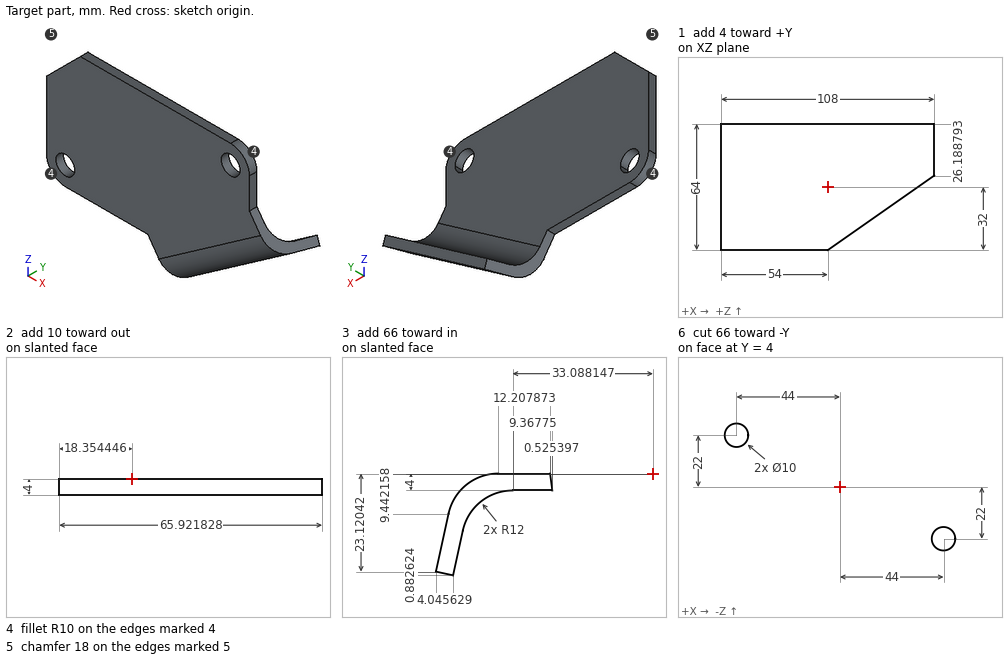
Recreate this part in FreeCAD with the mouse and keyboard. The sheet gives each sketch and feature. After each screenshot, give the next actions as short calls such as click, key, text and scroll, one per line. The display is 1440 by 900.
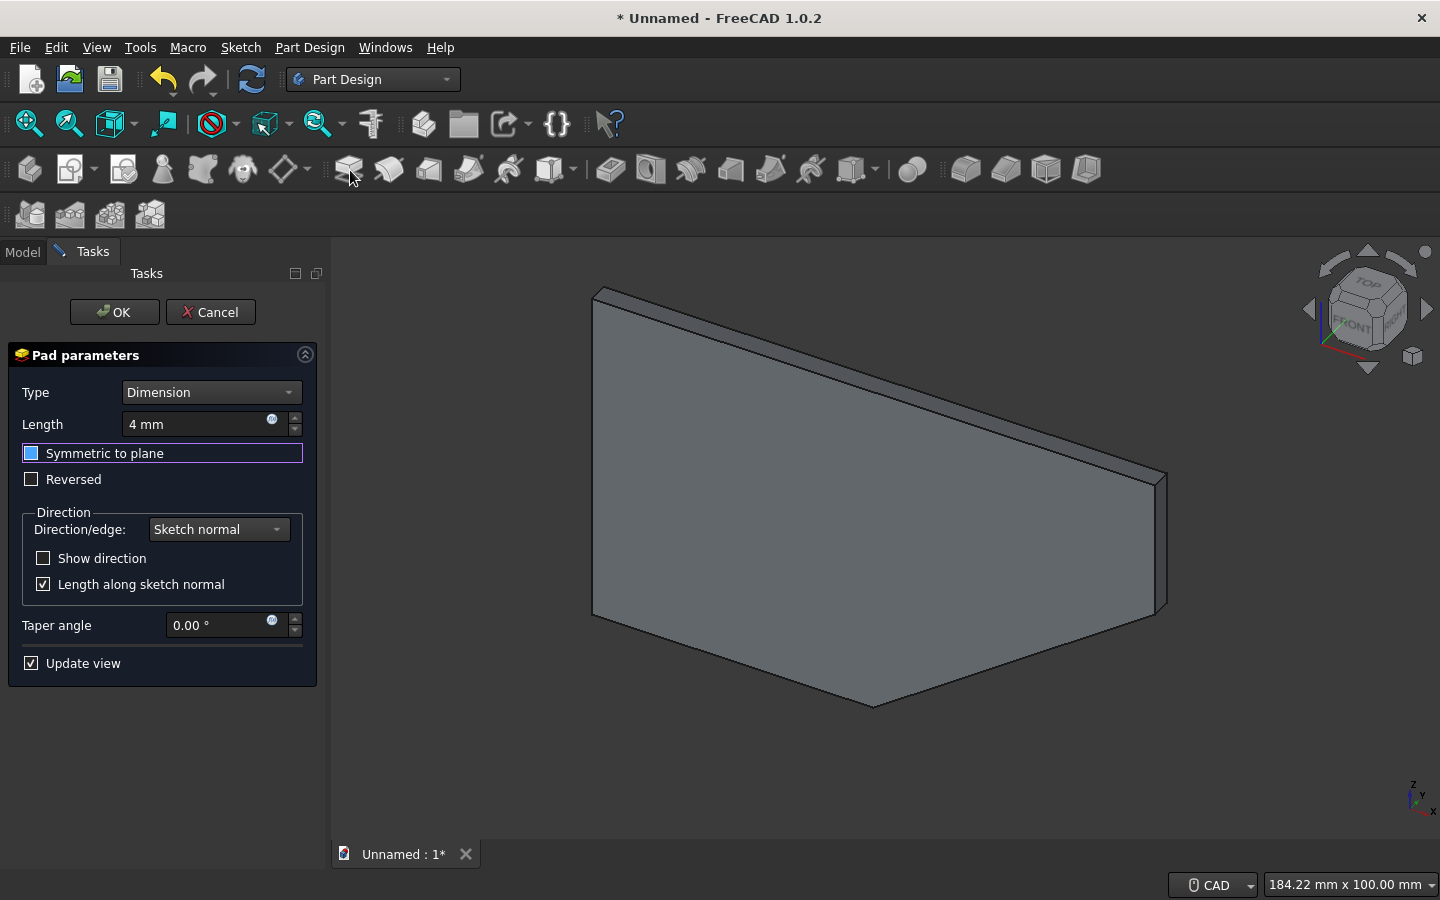
click(30, 479)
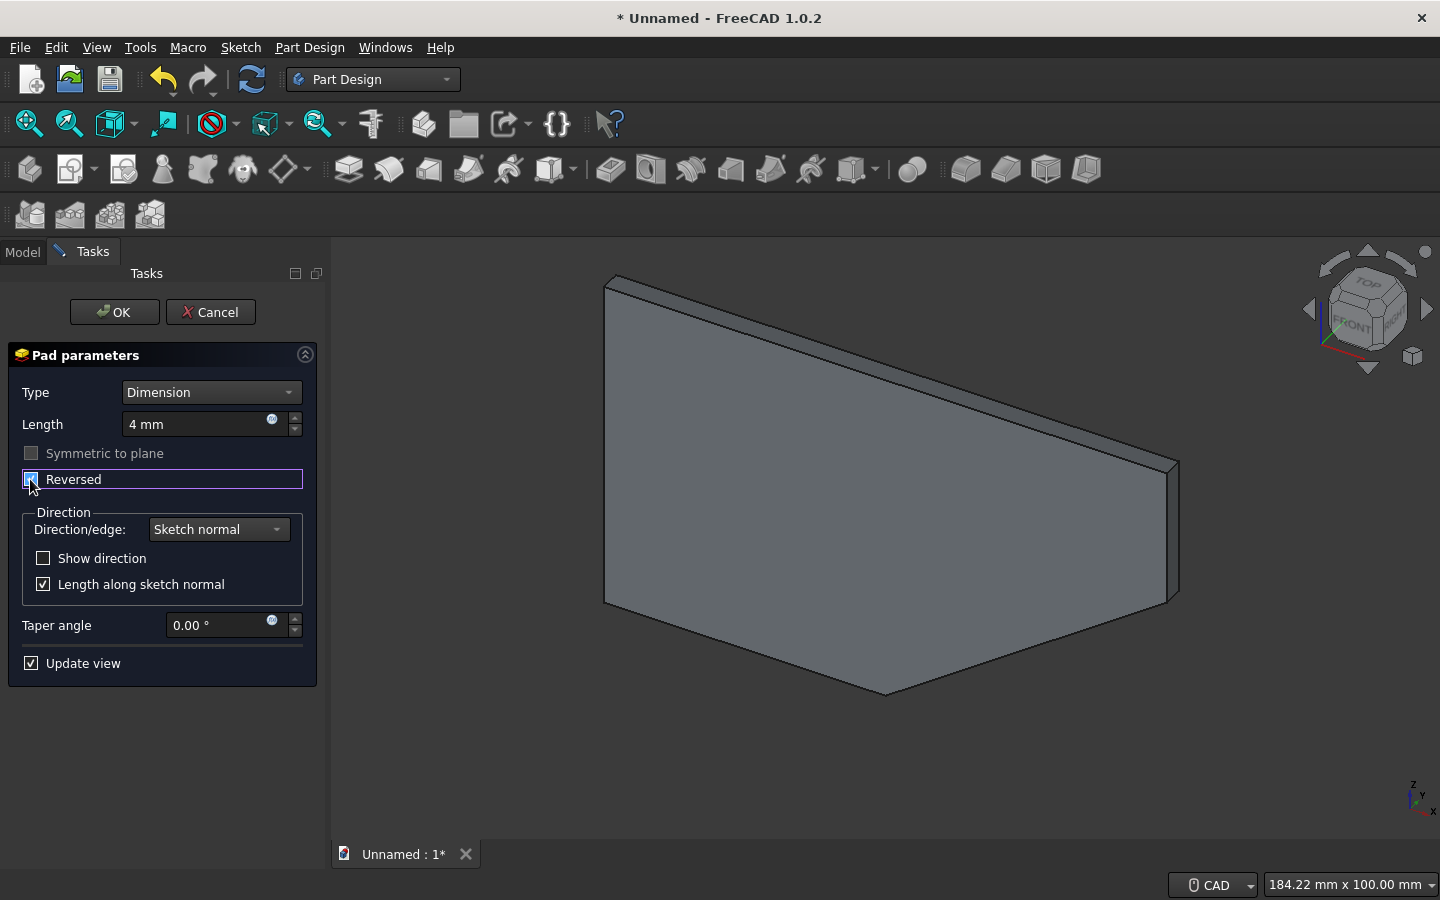
click(115, 312)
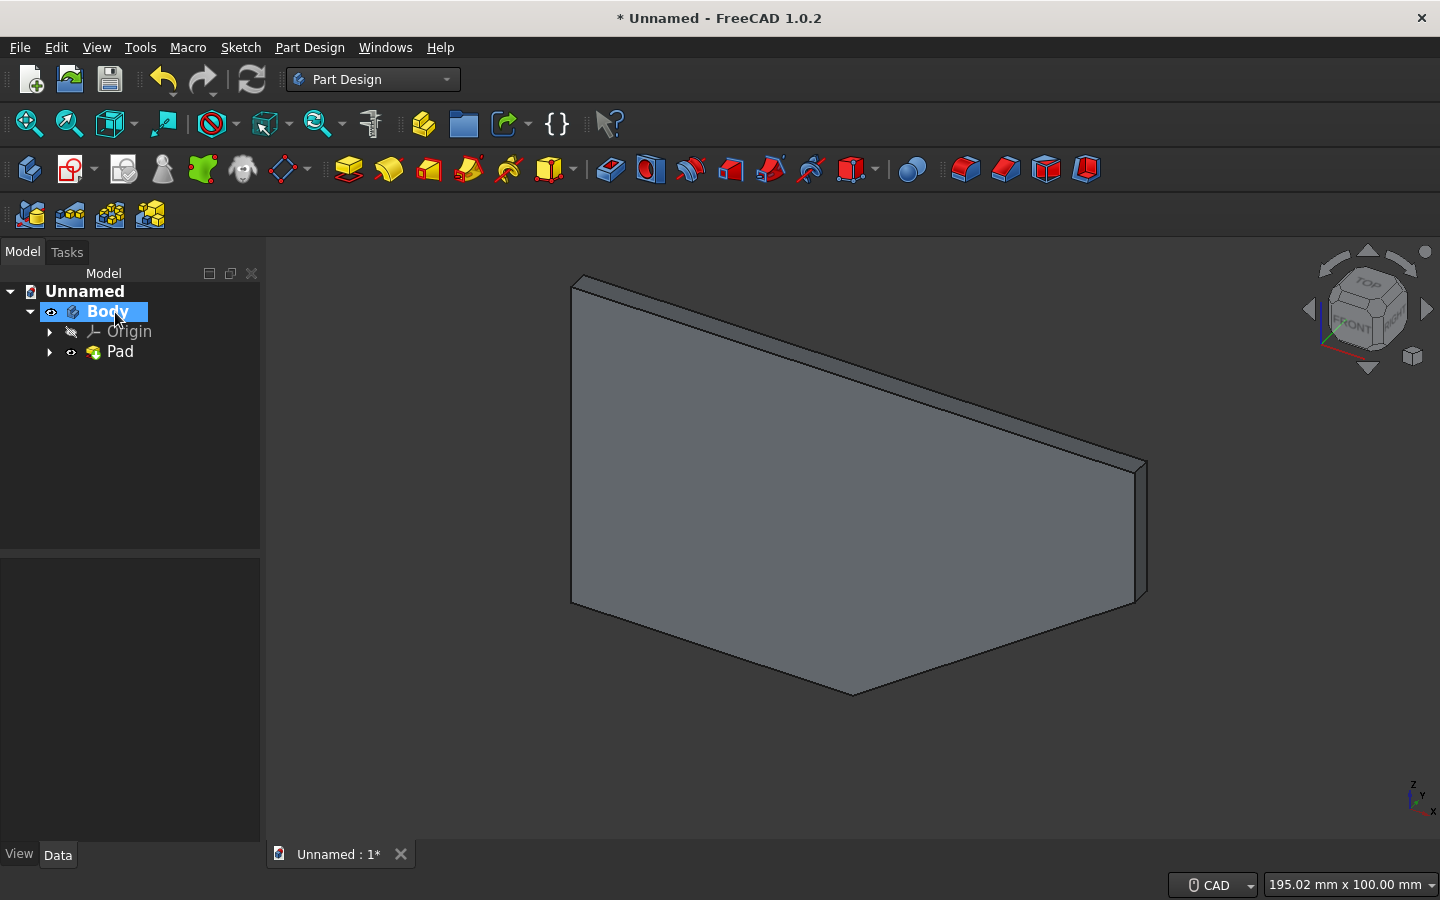
key(5)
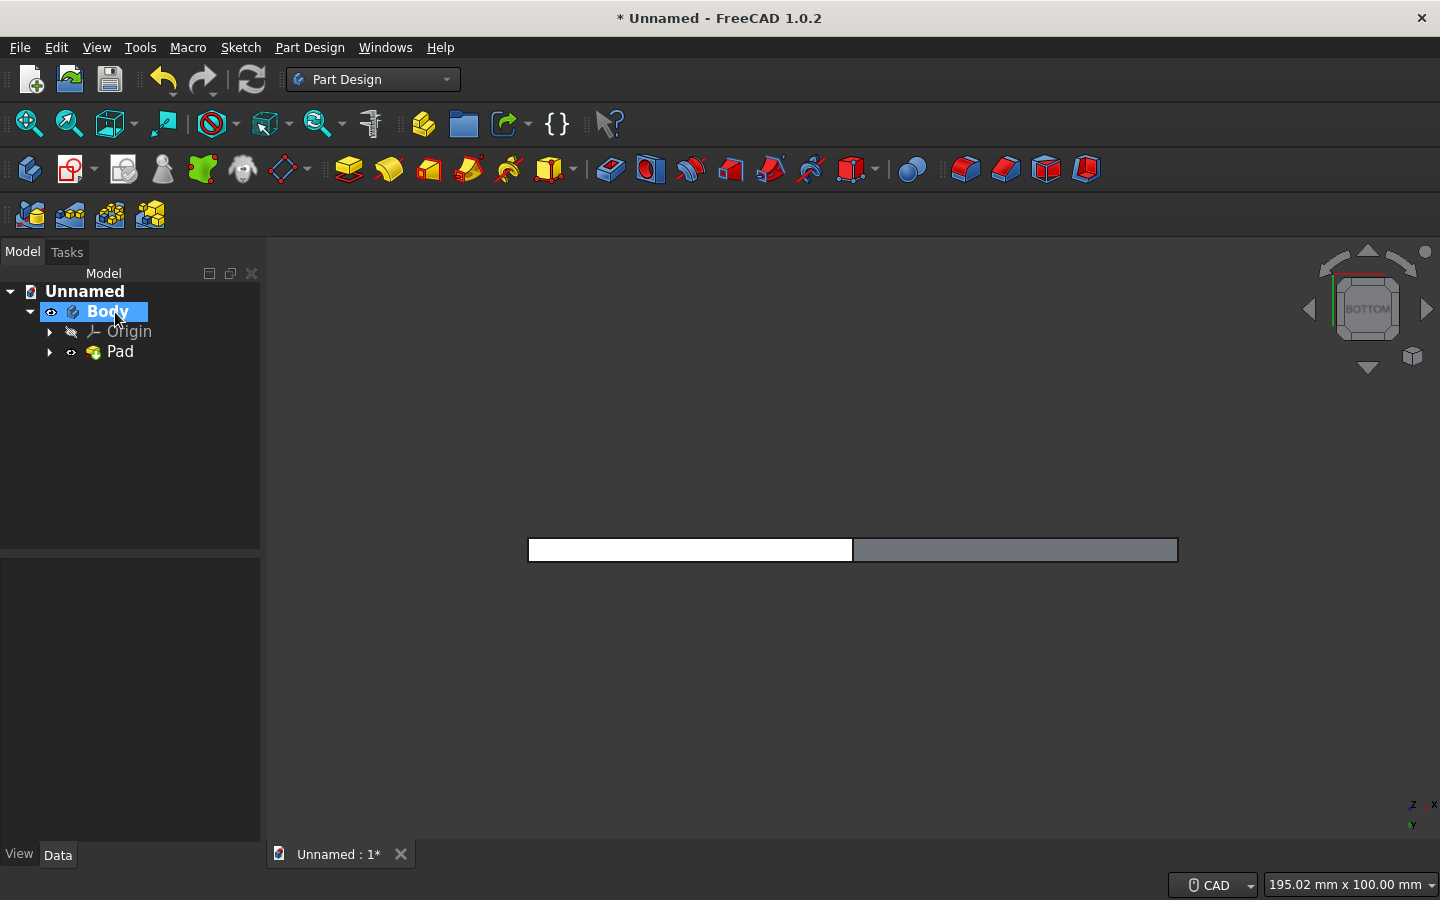
click(1155, 549)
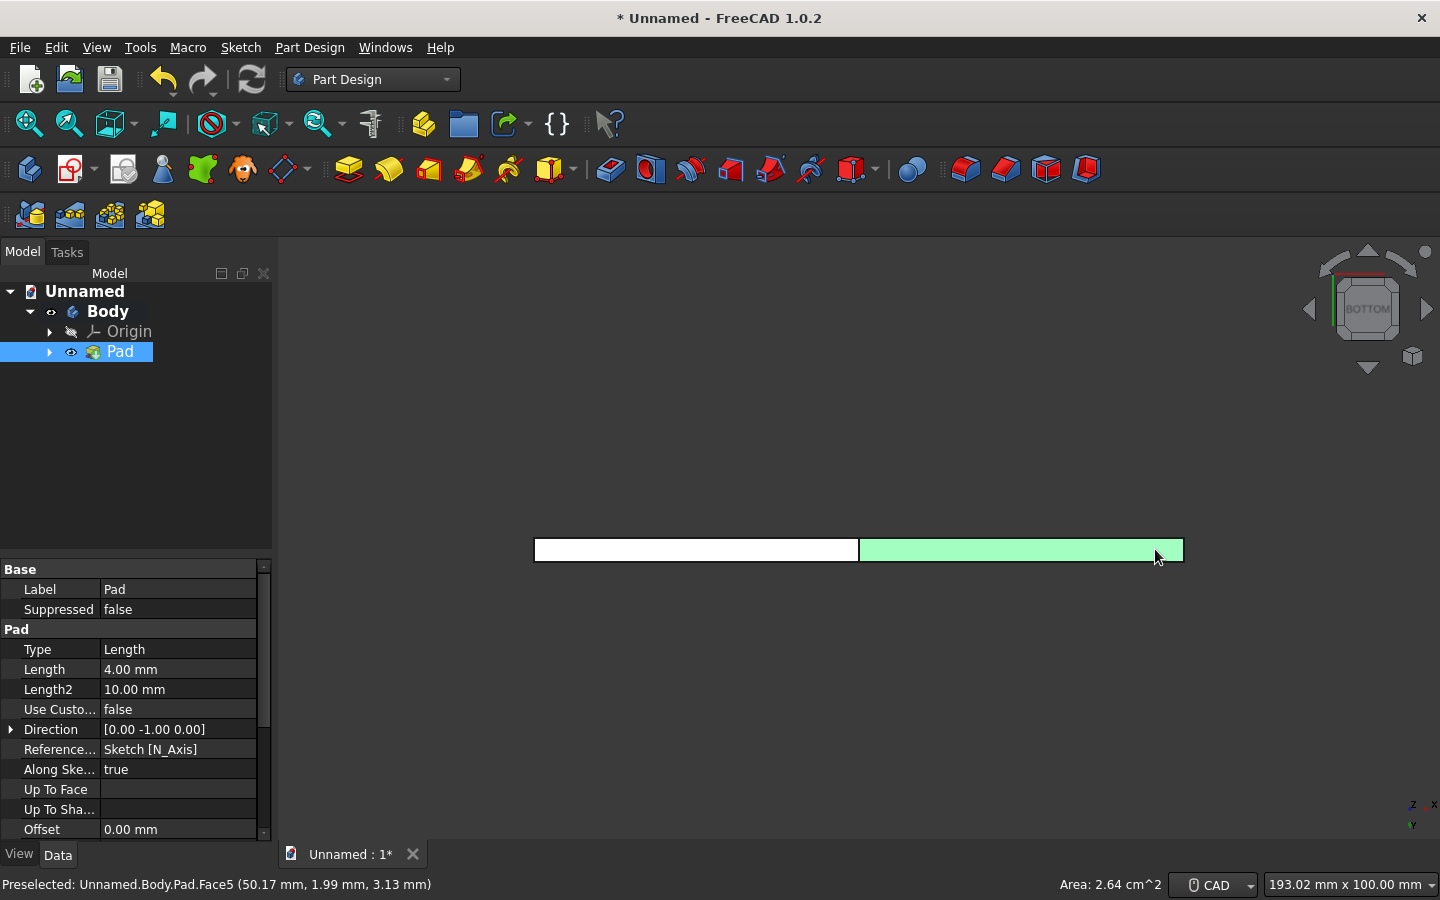
click(70, 170)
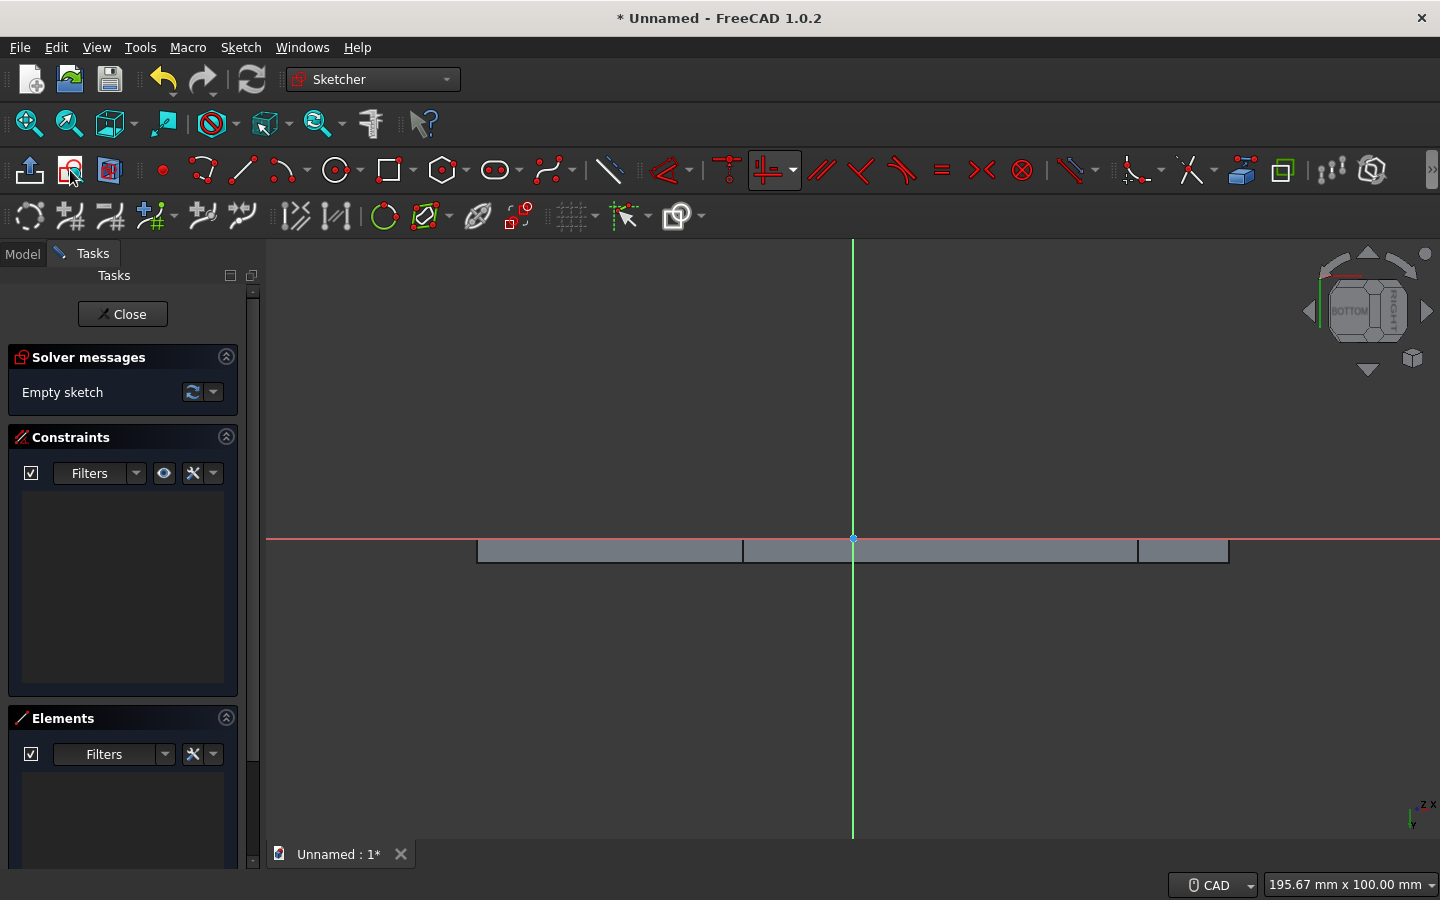
scroll(1131, 566, up, 3)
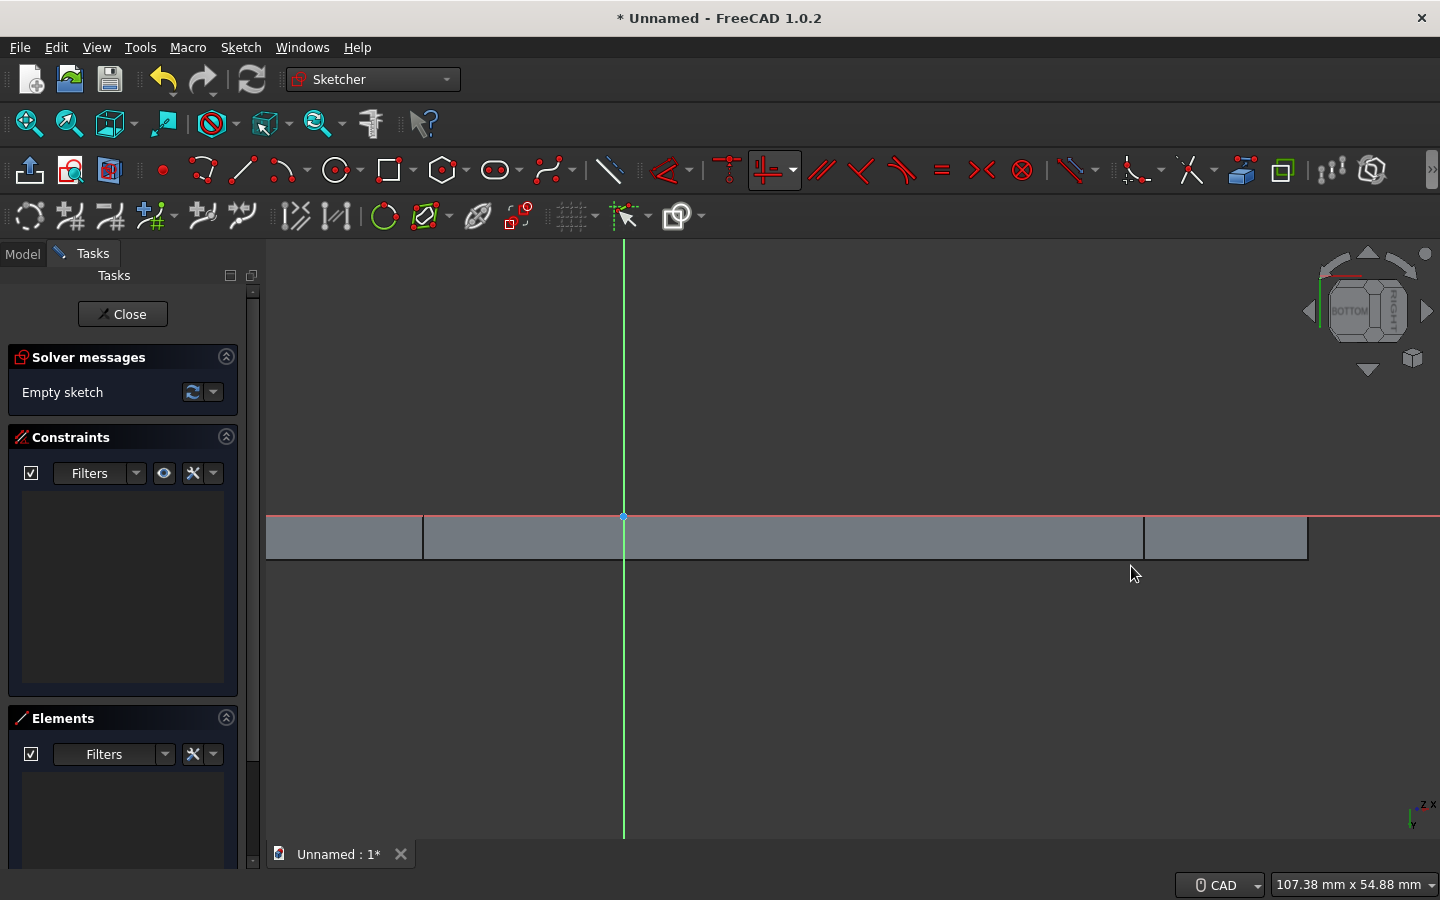
key(g)
key(r)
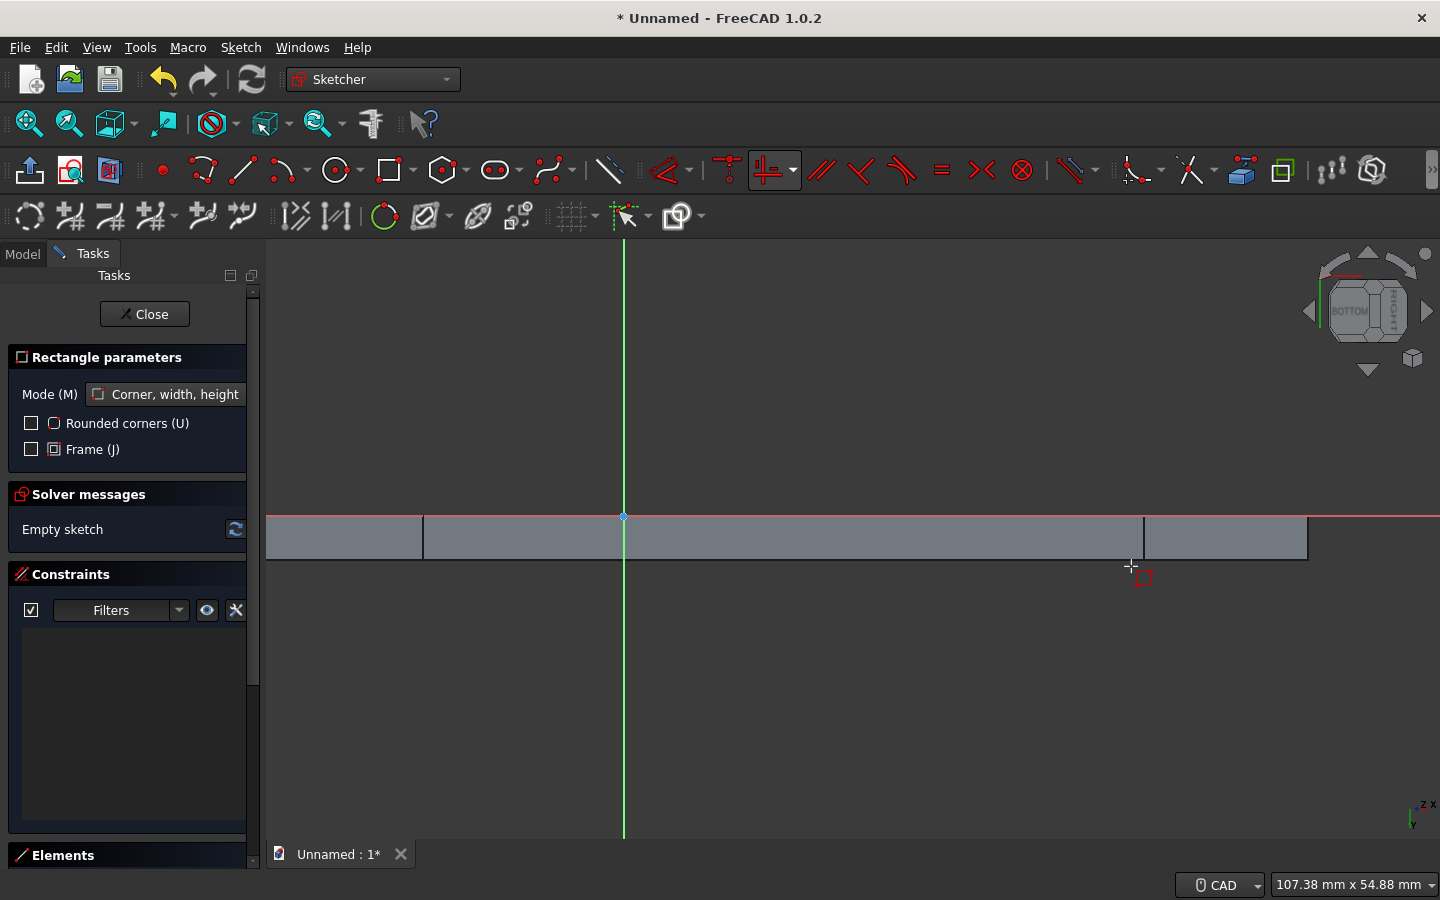
click(423, 516)
click(1144, 560)
key(Escape)